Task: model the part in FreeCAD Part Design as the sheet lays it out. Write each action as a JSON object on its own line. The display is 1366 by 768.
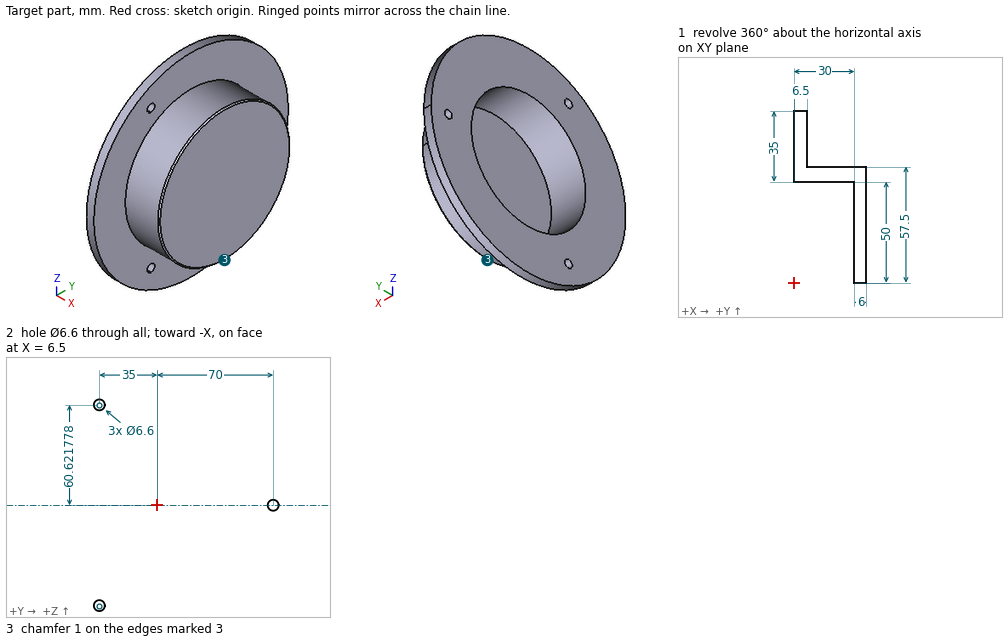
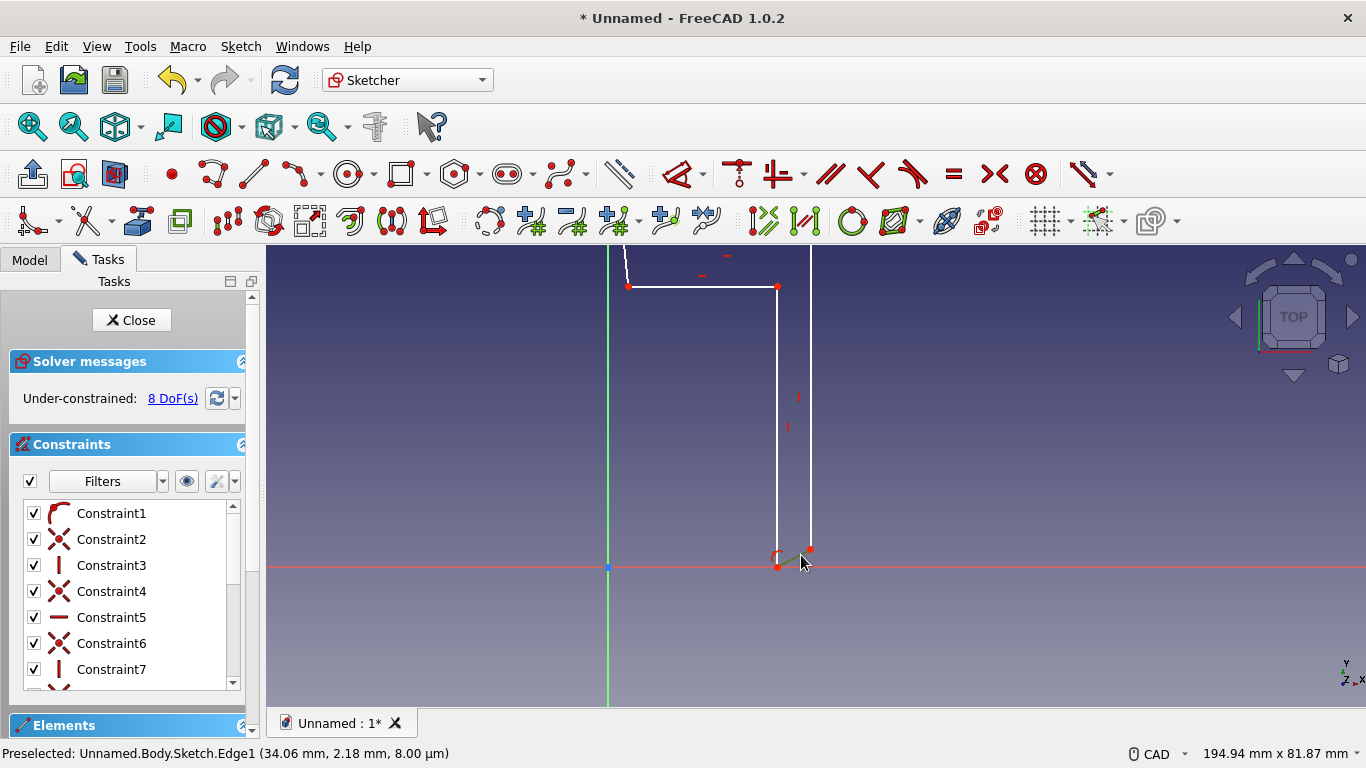
{"action": "left_click", "coordinate": [804, 174]}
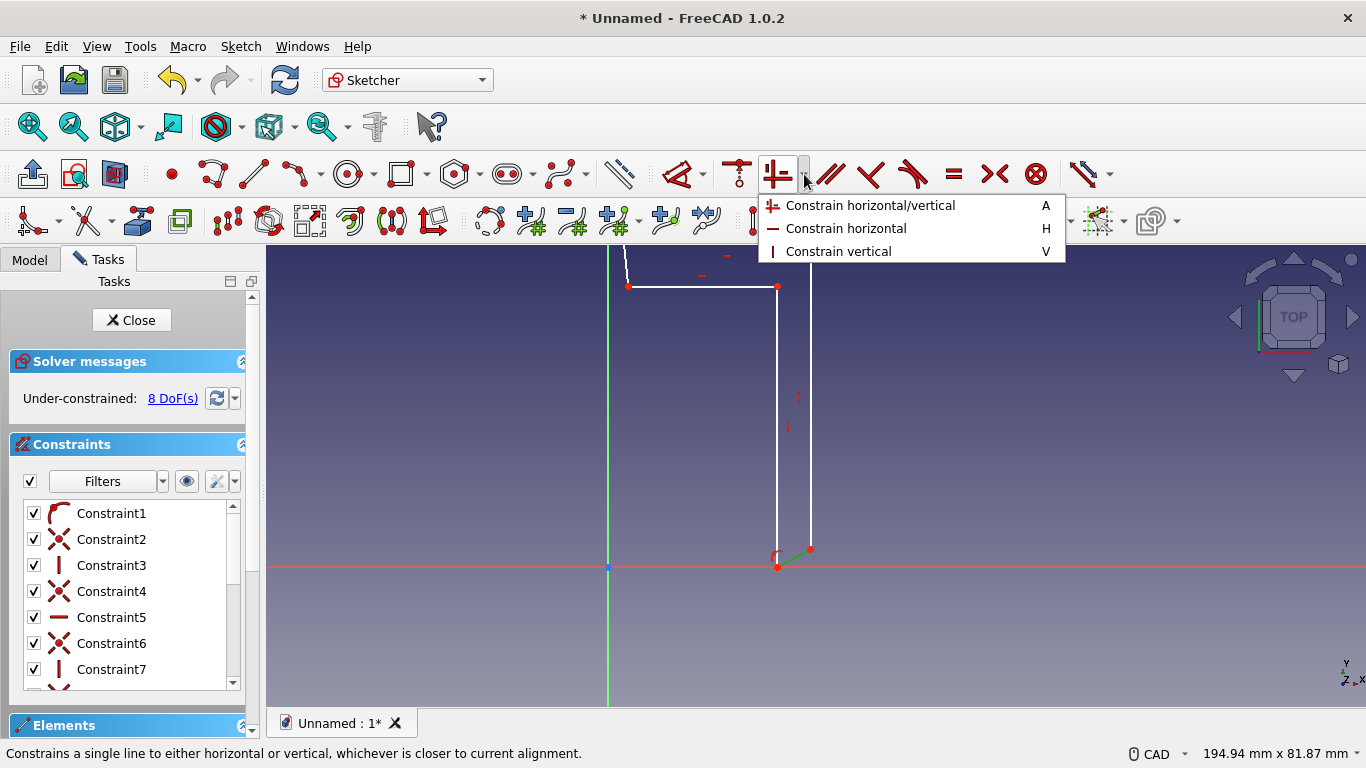
{"action": "left_click", "coordinate": [912, 228]}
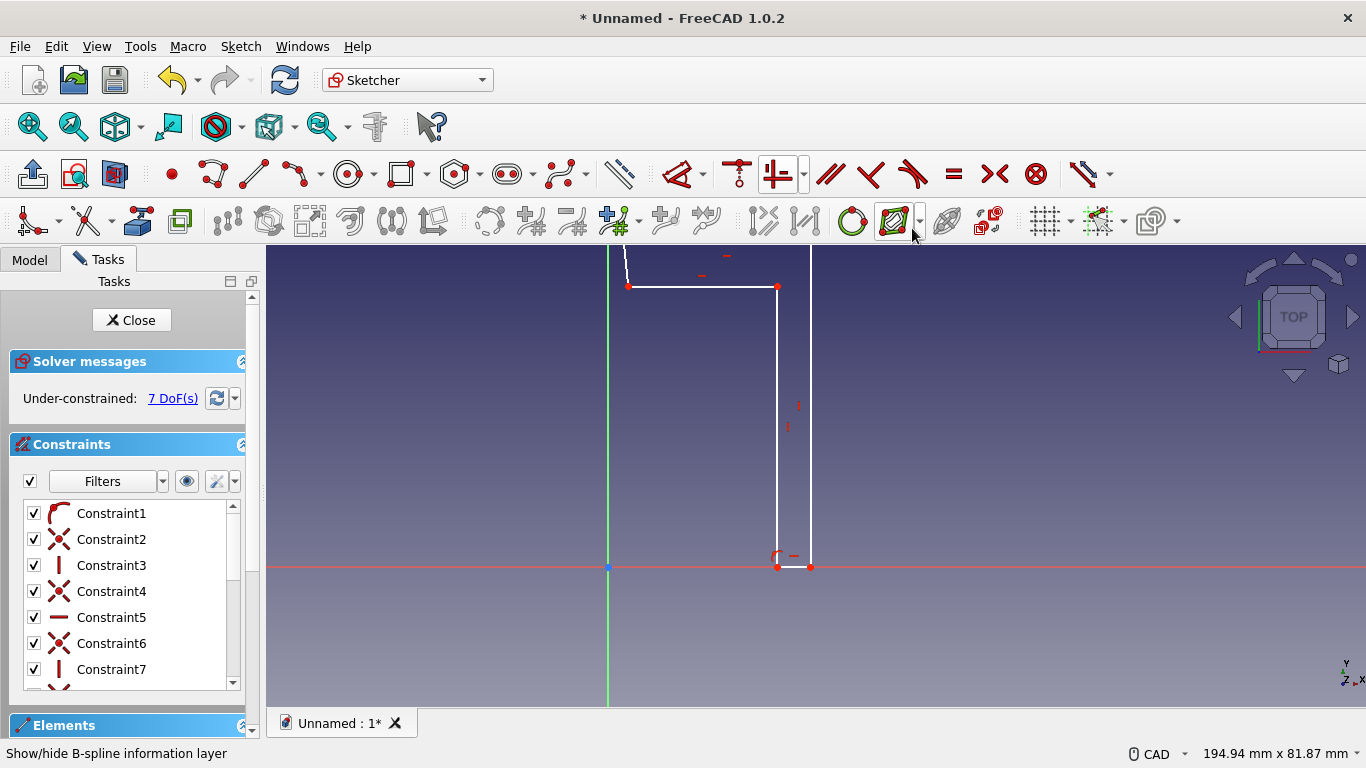
{"action": "scroll", "coordinate": [793, 657], "scroll_direction": "down", "scroll_amount": 3}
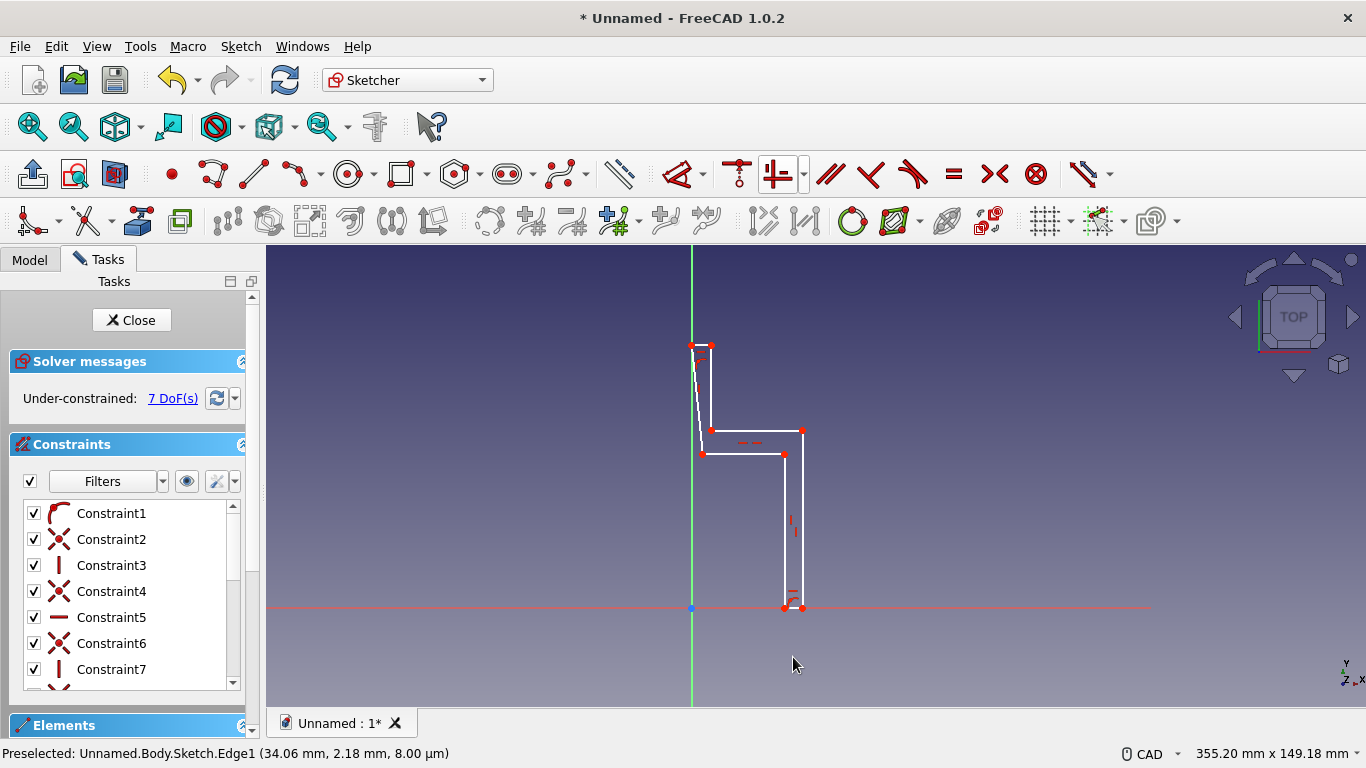
{"action": "scroll", "coordinate": [700, 422], "scroll_direction": "up", "scroll_amount": 3}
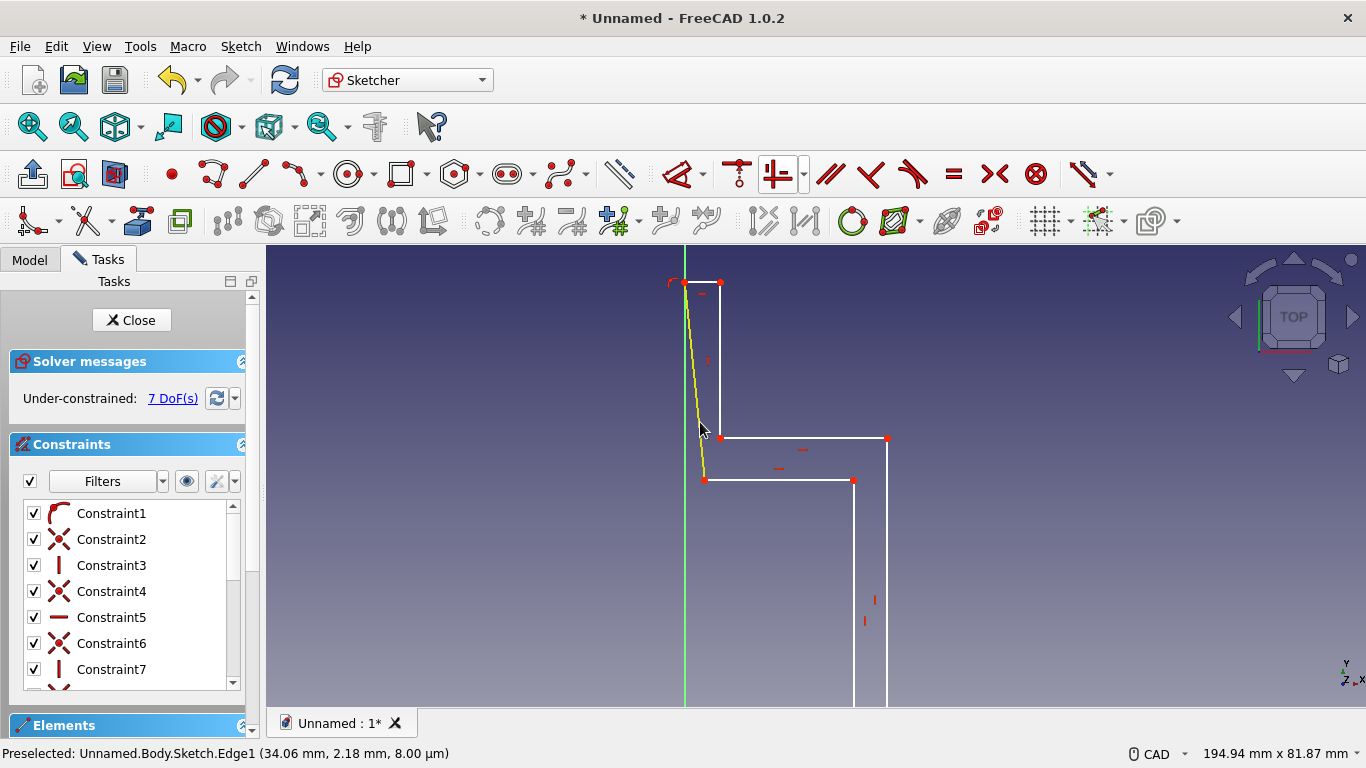
{"action": "left_click", "coordinate": [699, 421]}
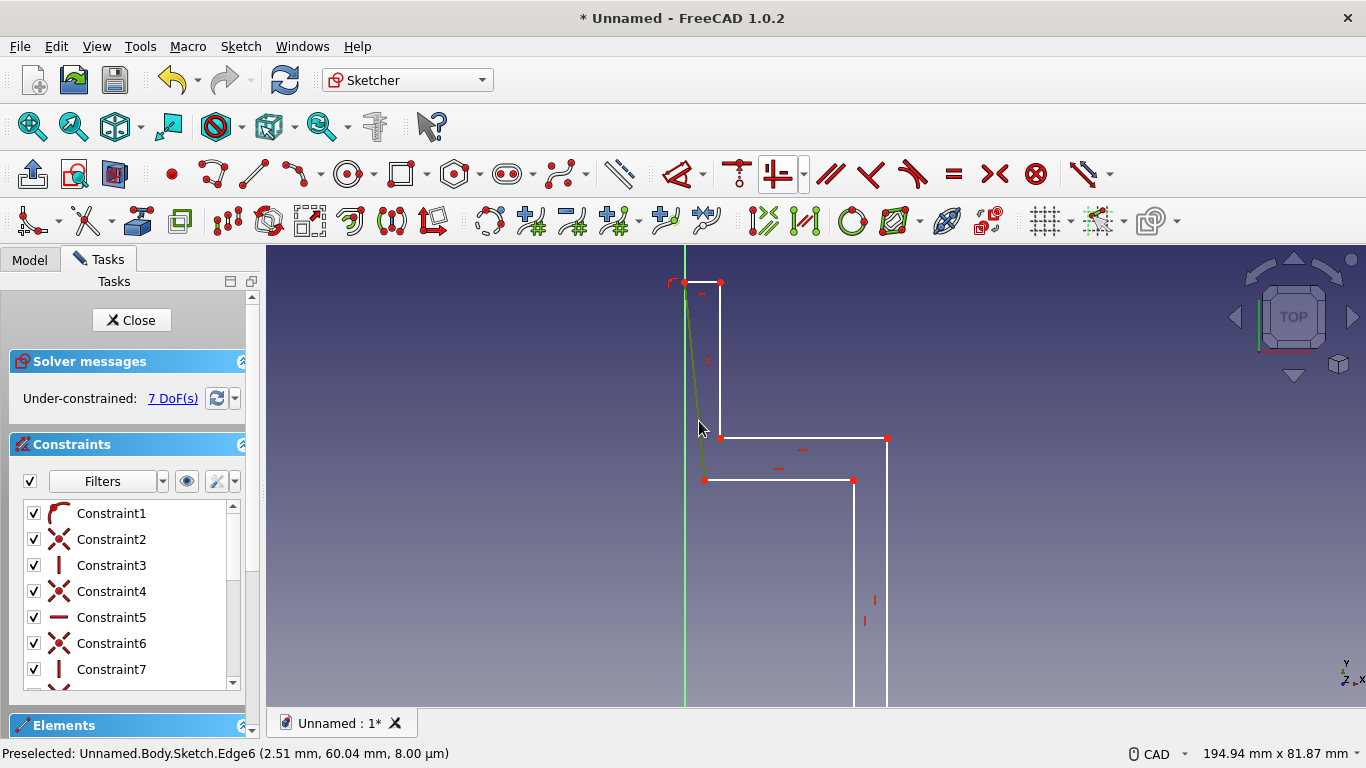
{"action": "left_click", "coordinate": [804, 174]}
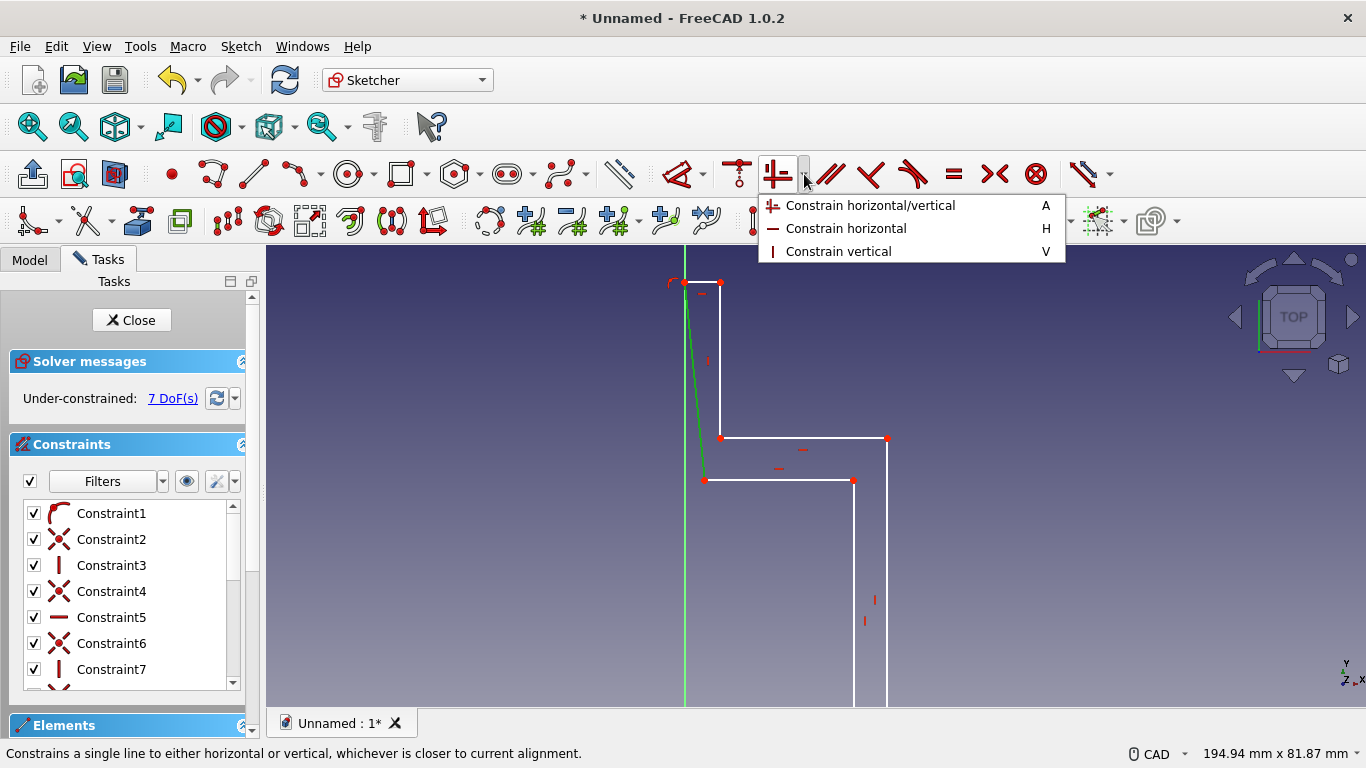
{"action": "left_click", "coordinate": [912, 252]}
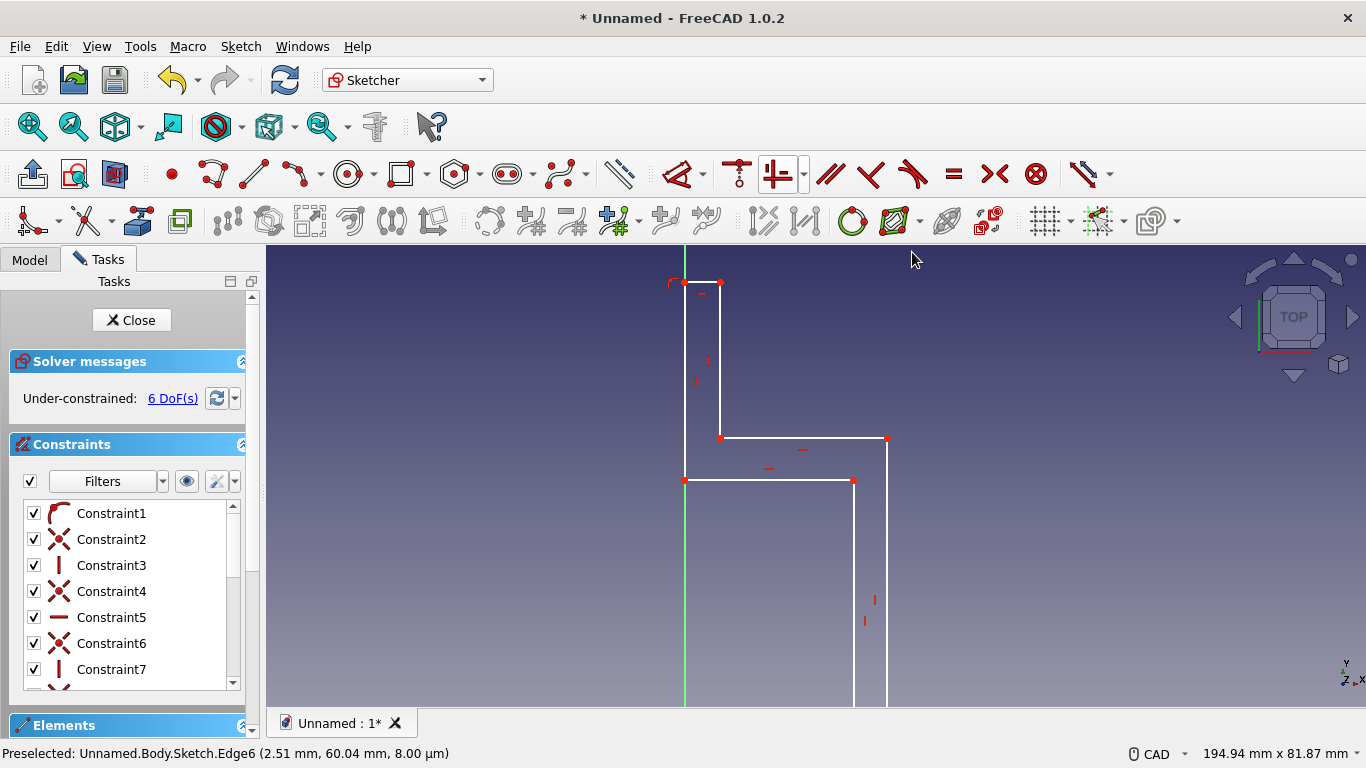
{"action": "scroll", "coordinate": [700, 421], "scroll_direction": "down", "scroll_amount": 3}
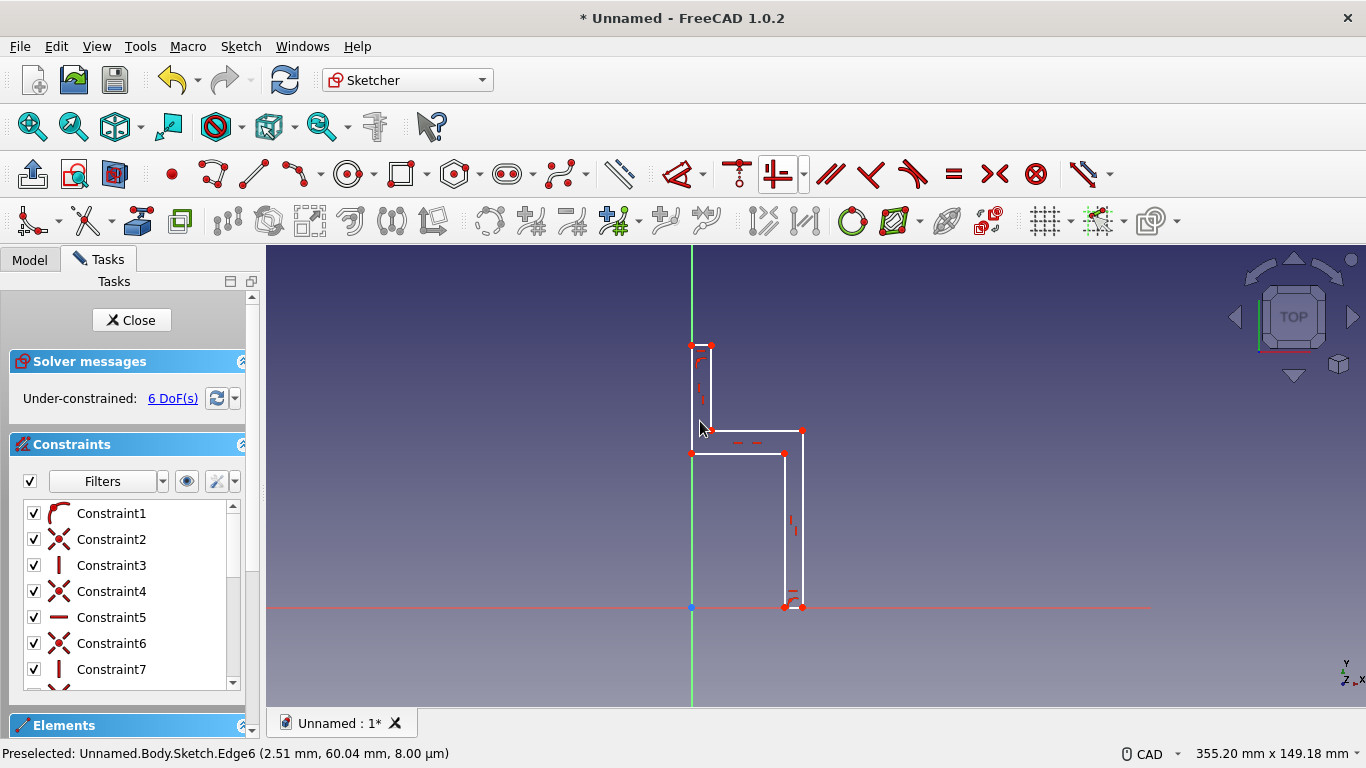
{"action": "scroll", "coordinate": [790, 608], "scroll_direction": "up", "scroll_amount": 5}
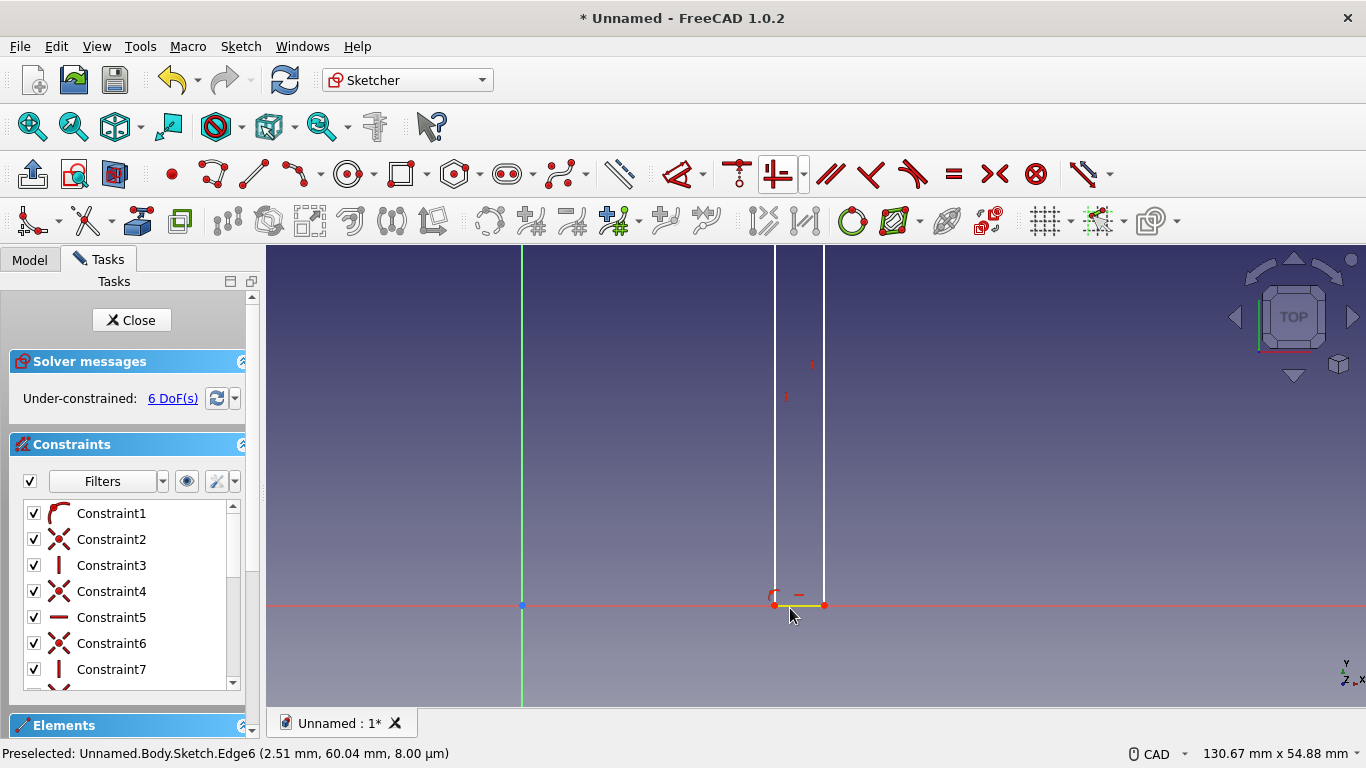
{"action": "left_click", "coordinate": [790, 606]}